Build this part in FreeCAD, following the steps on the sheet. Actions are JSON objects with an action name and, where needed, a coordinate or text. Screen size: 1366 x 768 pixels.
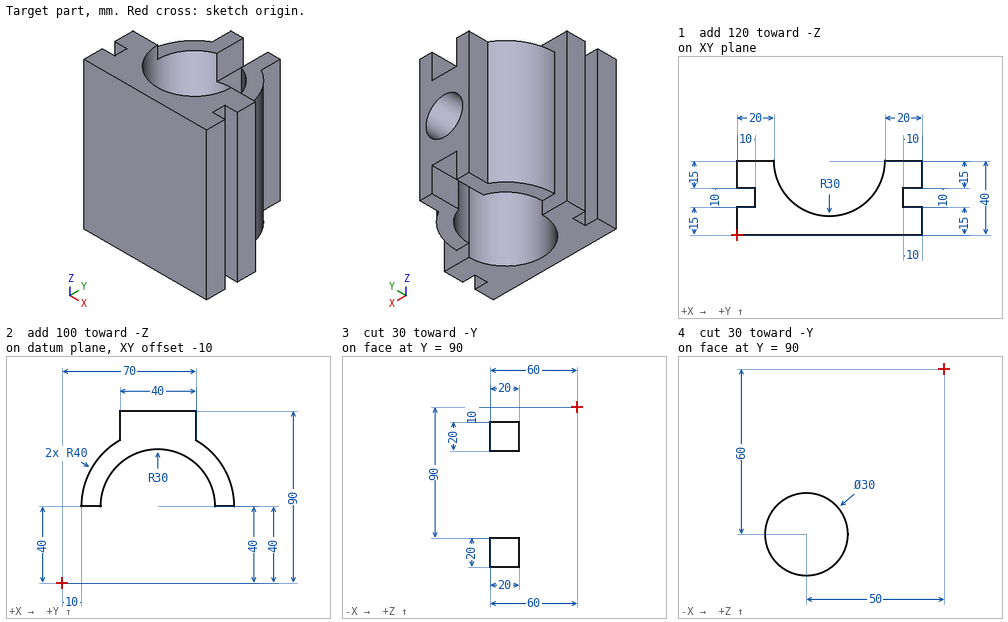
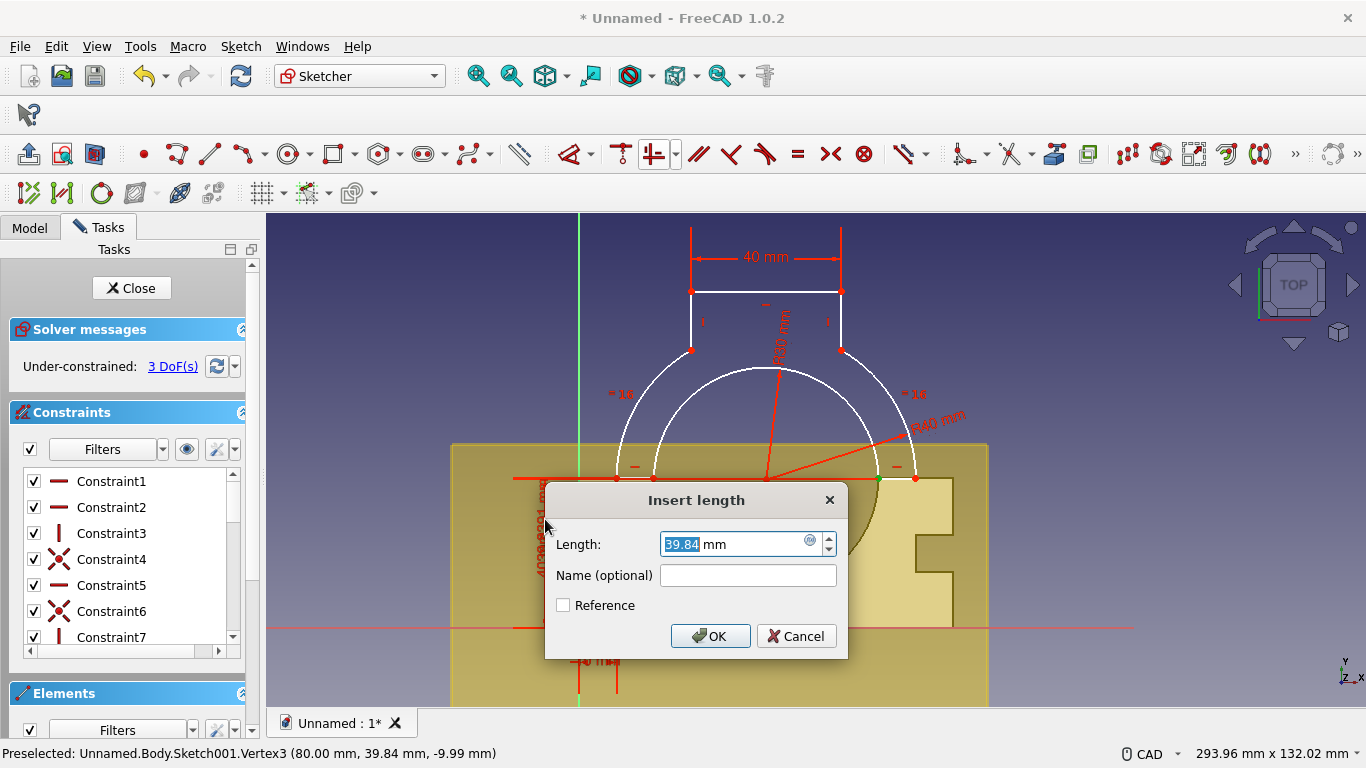
{"action": "type", "text": "40"}
{"action": "key", "text": "Return"}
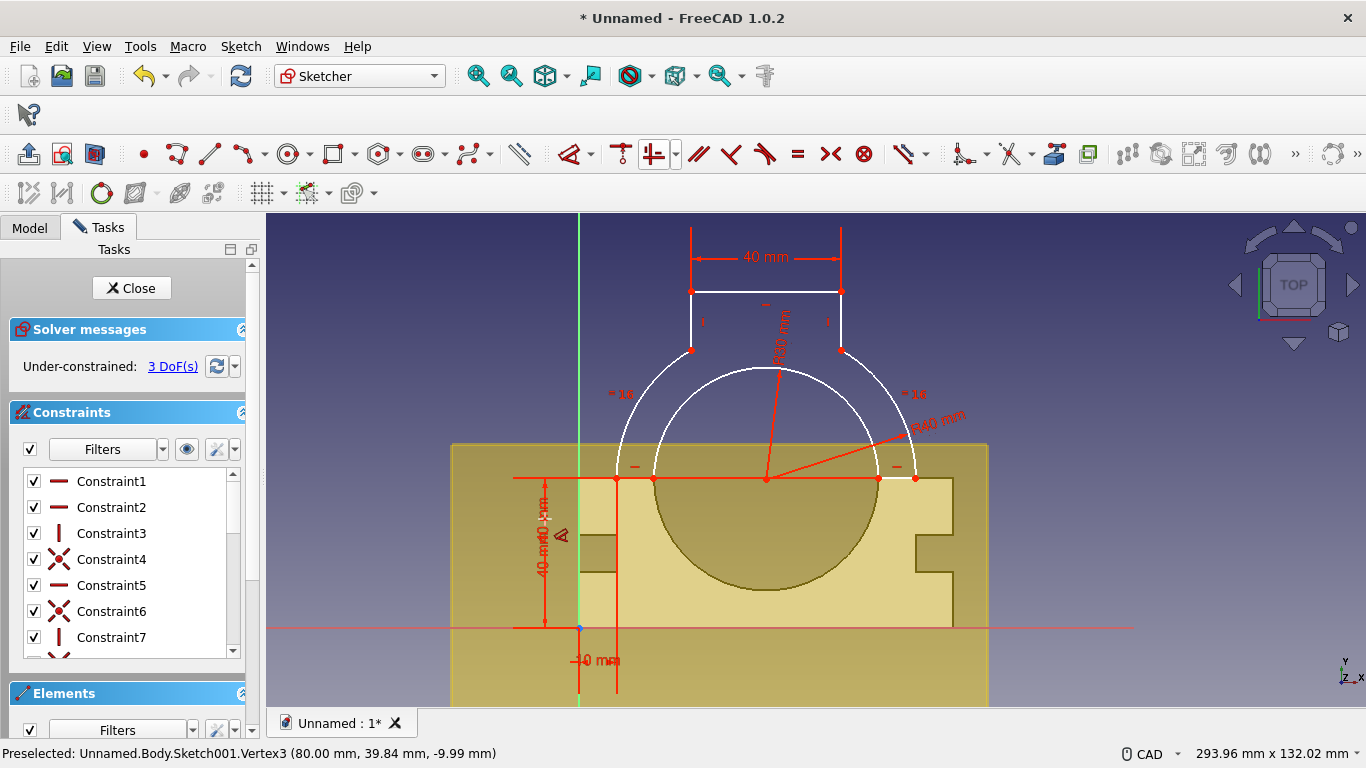
{"action": "left_click", "coordinate": [841, 350]}
{"action": "left_click", "coordinate": [710, 662]}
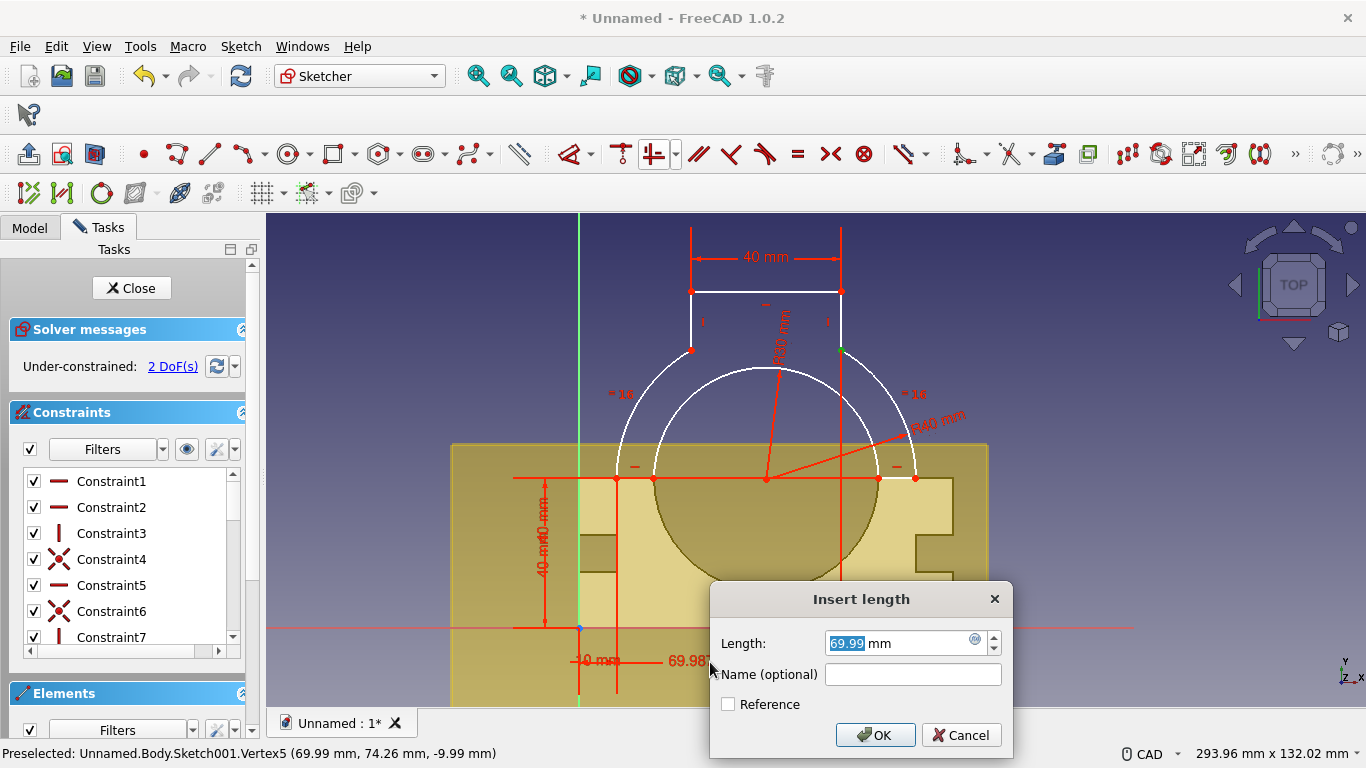
{"action": "type", "text": "70"}
{"action": "key", "text": "Return"}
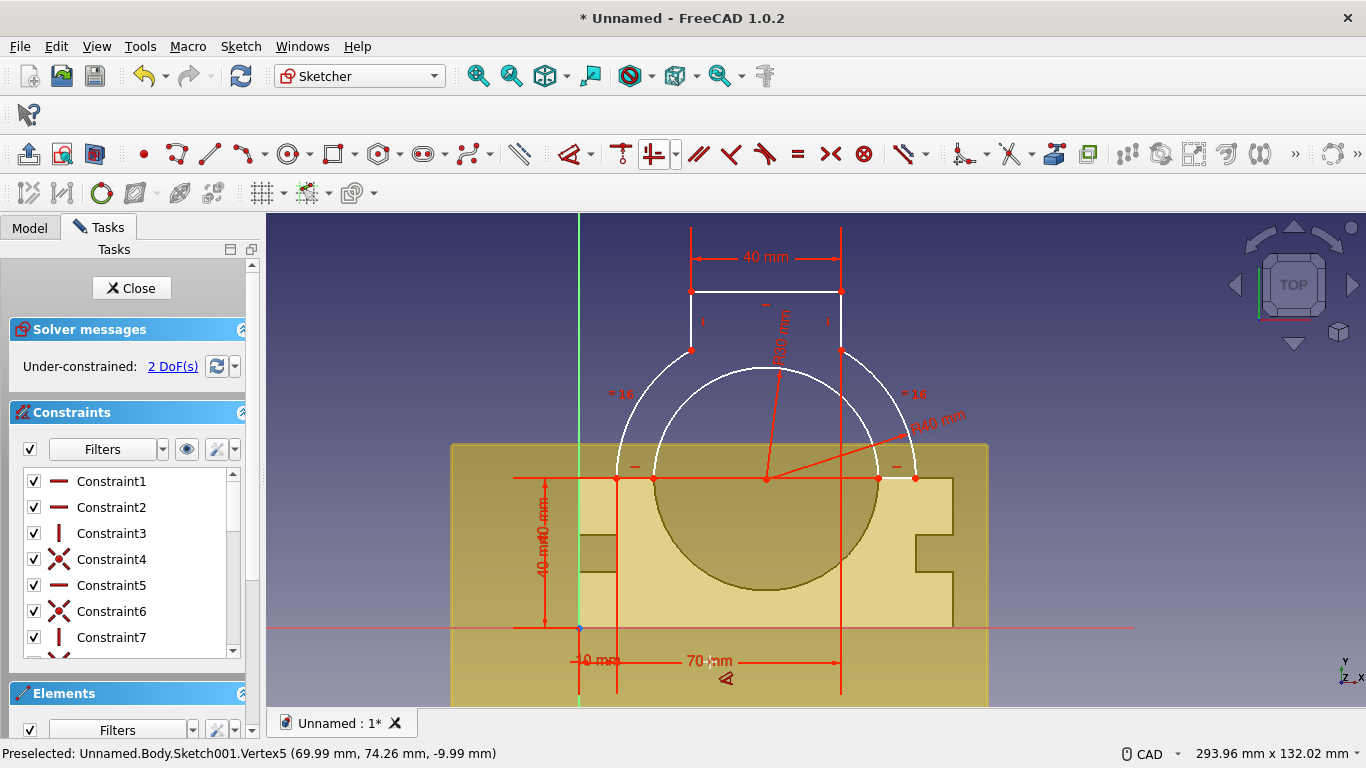
{"action": "left_click", "coordinate": [841, 292]}
{"action": "left_click", "coordinate": [545, 460]}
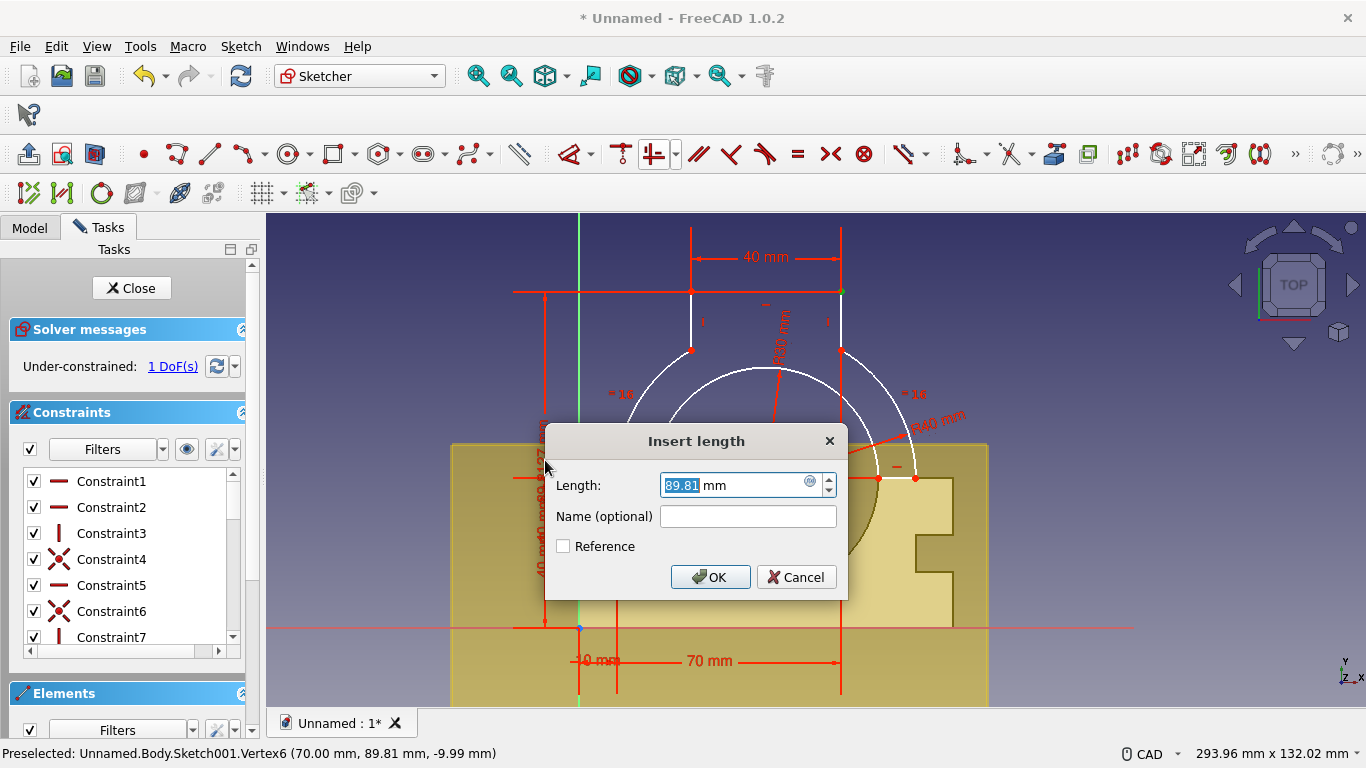
{"action": "type", "text": "90"}
{"action": "key", "text": "Return"}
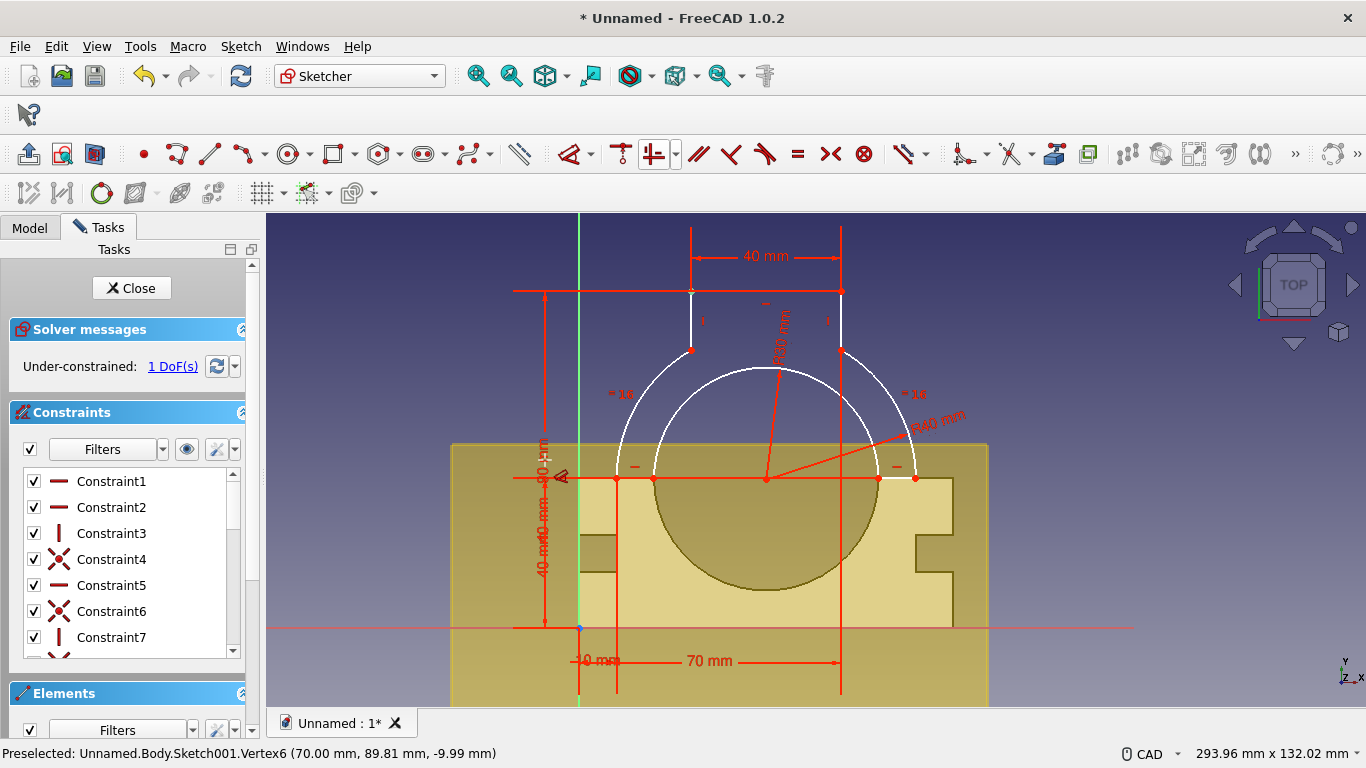
{"action": "left_click", "coordinate": [766, 480]}
{"action": "left_click", "coordinate": [545, 588]}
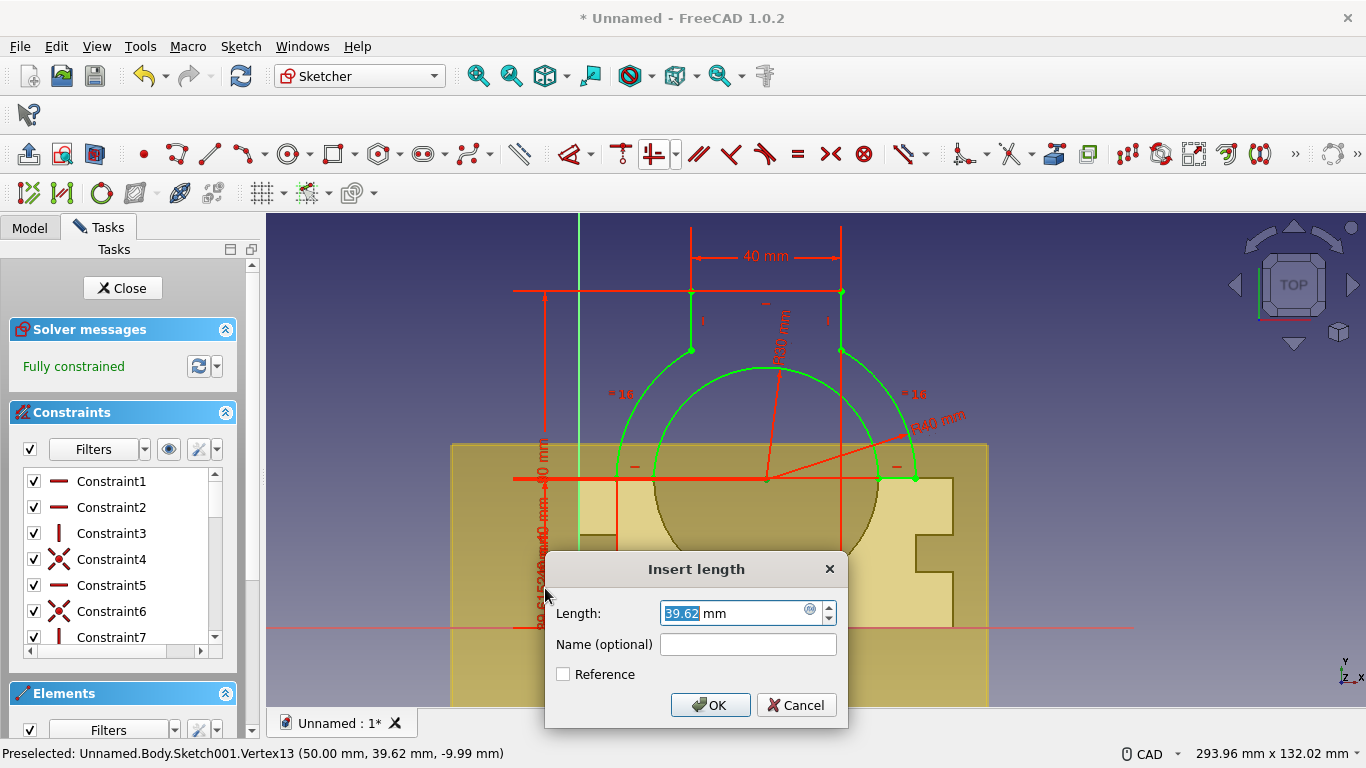
{"action": "type", "text": "40"}
{"action": "key", "text": "Return"}
{"action": "key", "text": "Escape"}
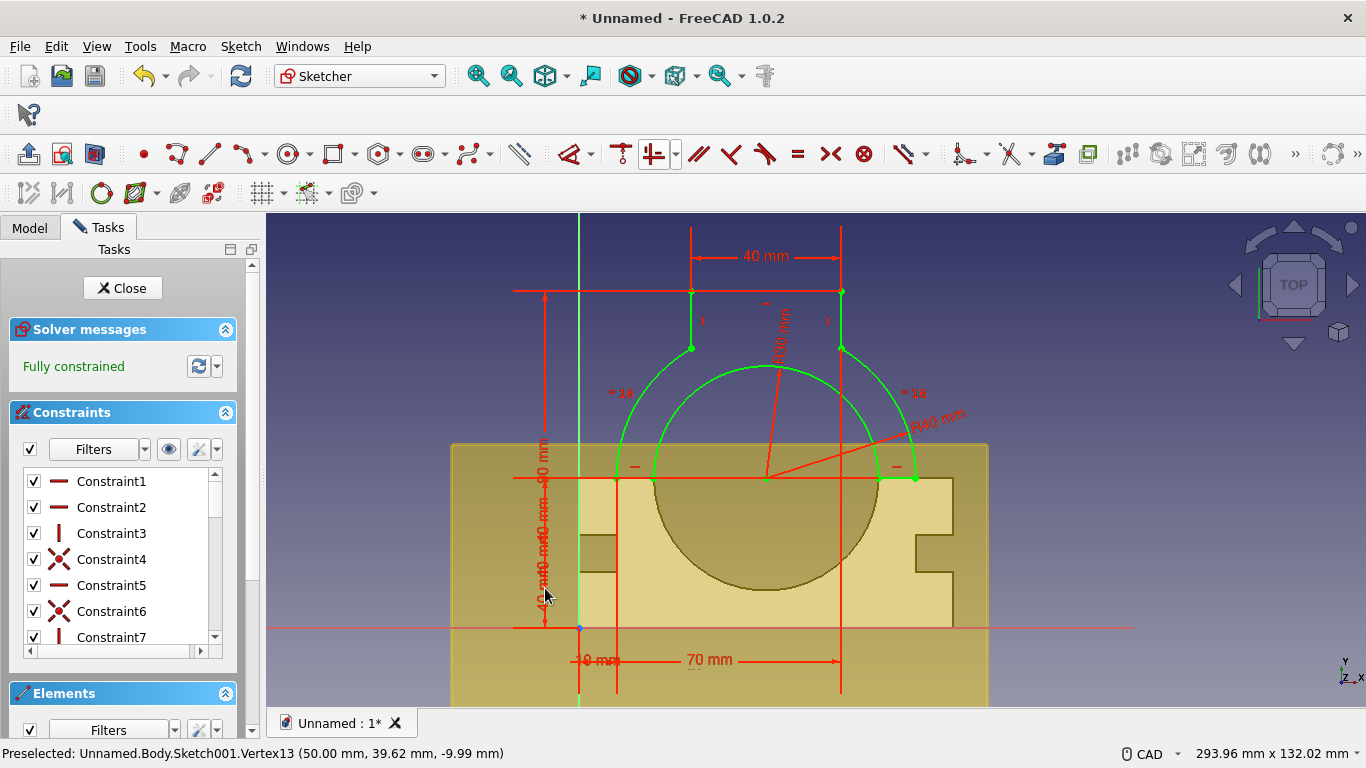
{"action": "left_click", "coordinate": [123, 288]}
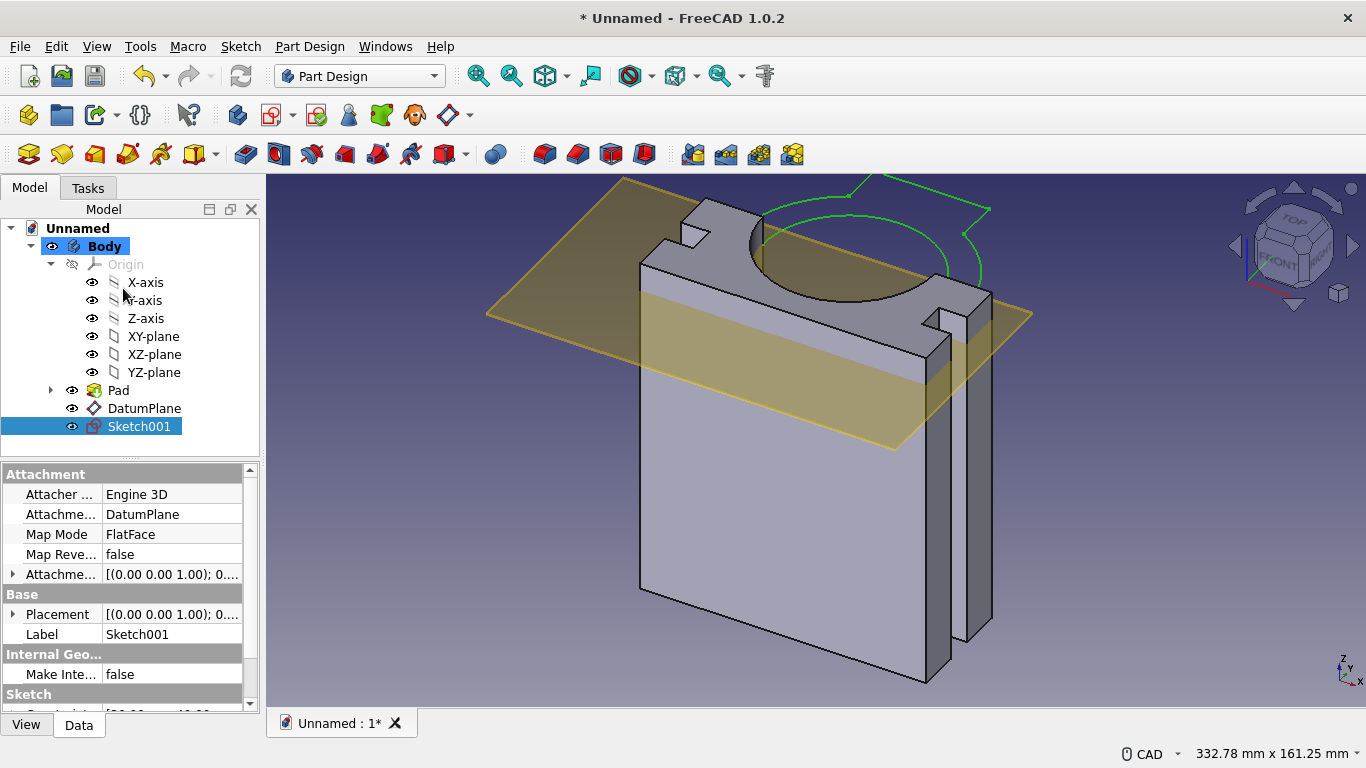
{"action": "left_click", "coordinate": [29, 154]}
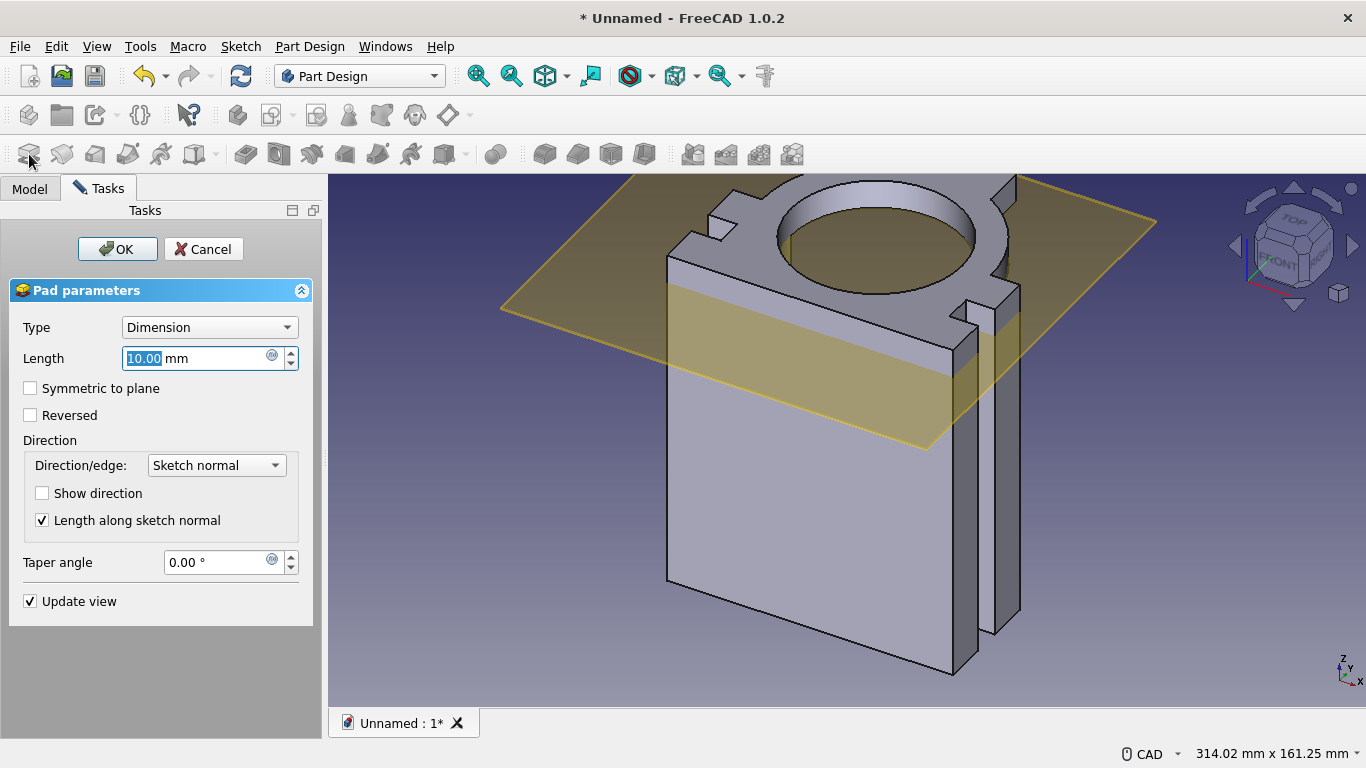
{"action": "type", "text": "100"}
{"action": "key", "text": "Tab"}